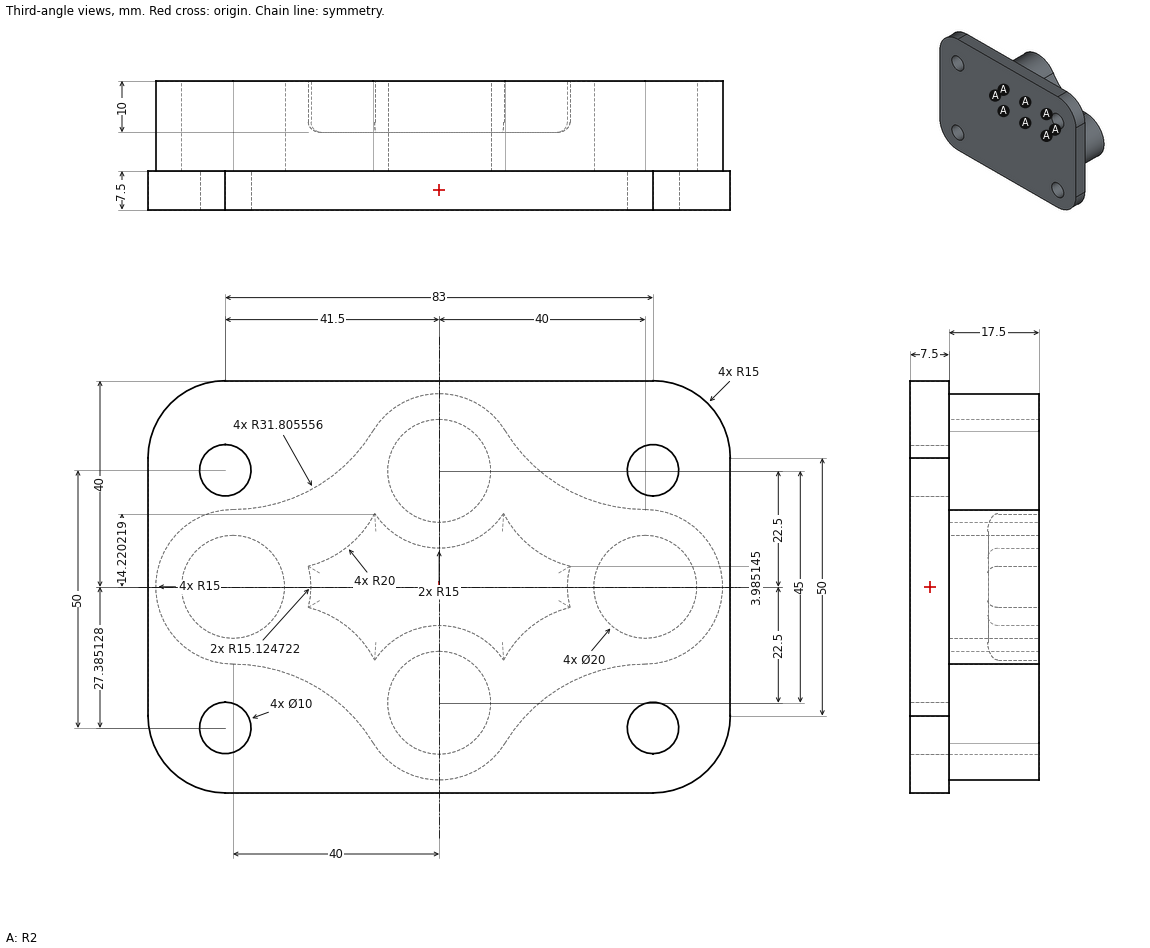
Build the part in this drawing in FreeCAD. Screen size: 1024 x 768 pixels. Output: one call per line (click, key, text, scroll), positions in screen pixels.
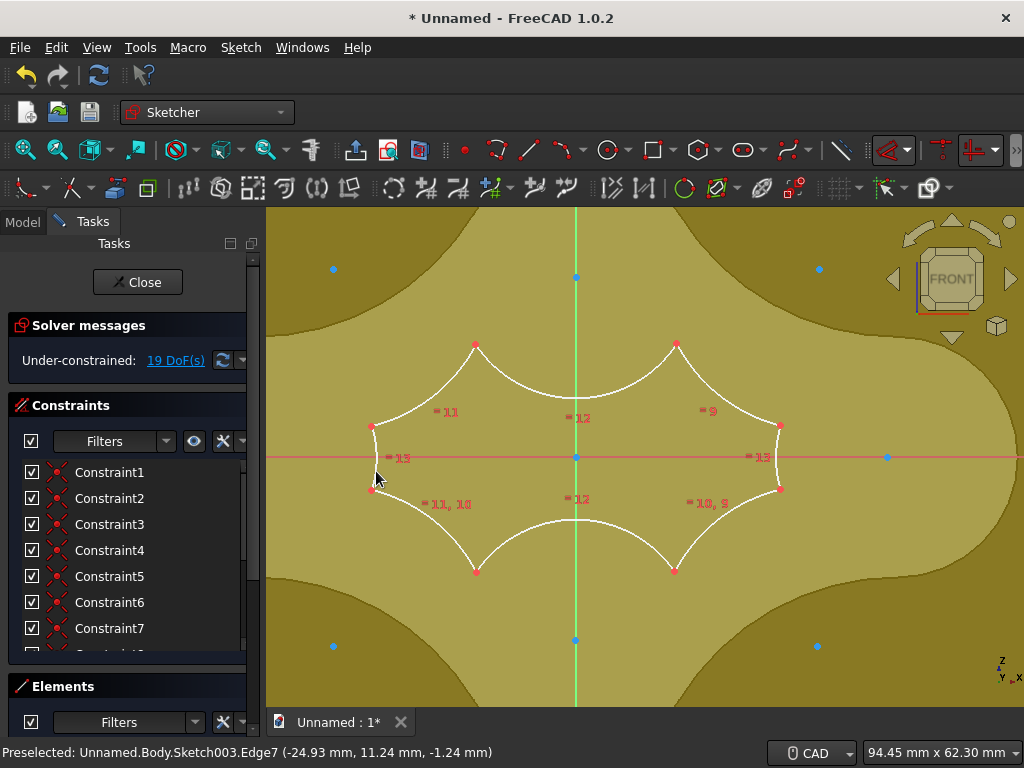
click(576, 278)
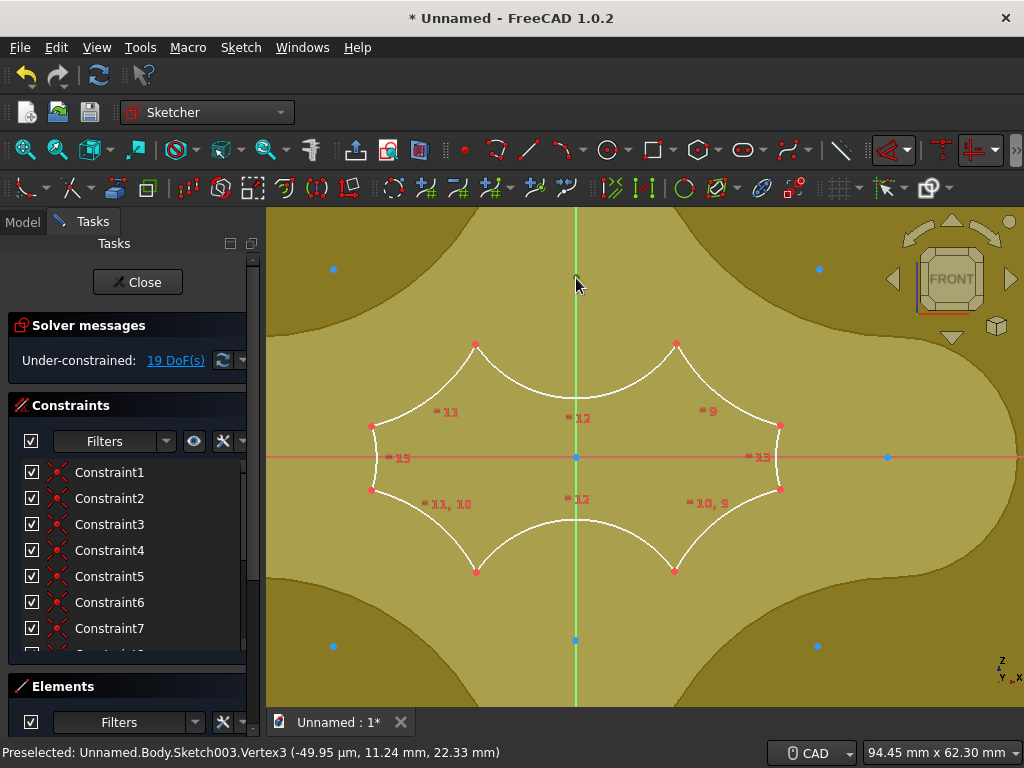
click(576, 647)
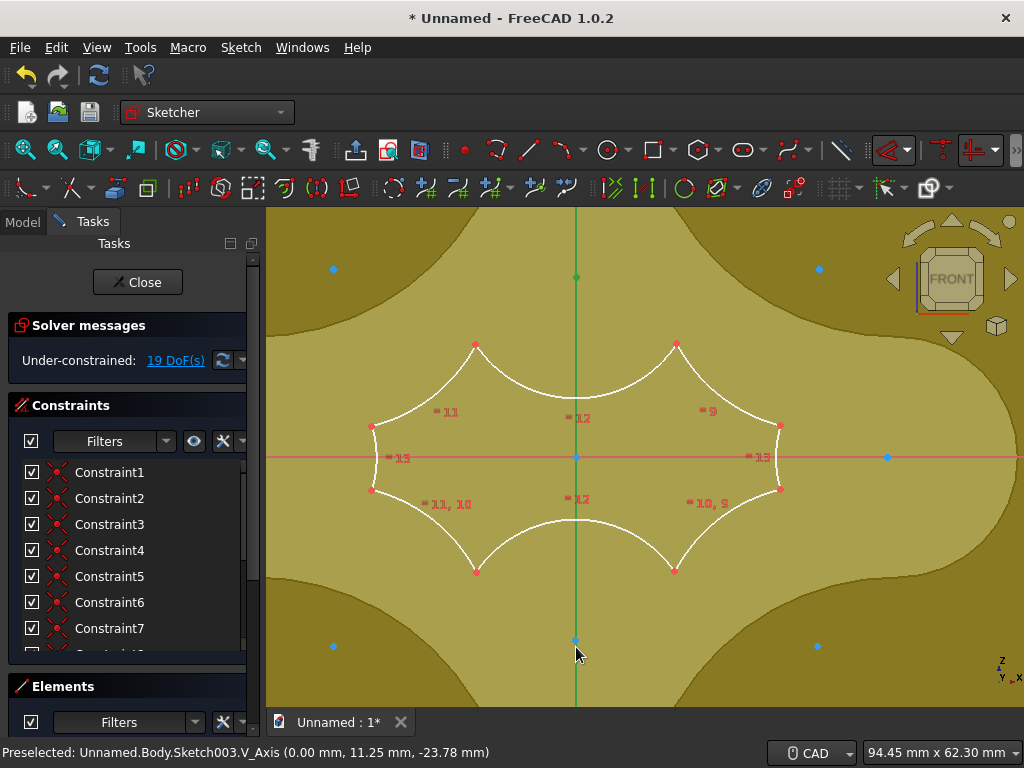
click(942, 150)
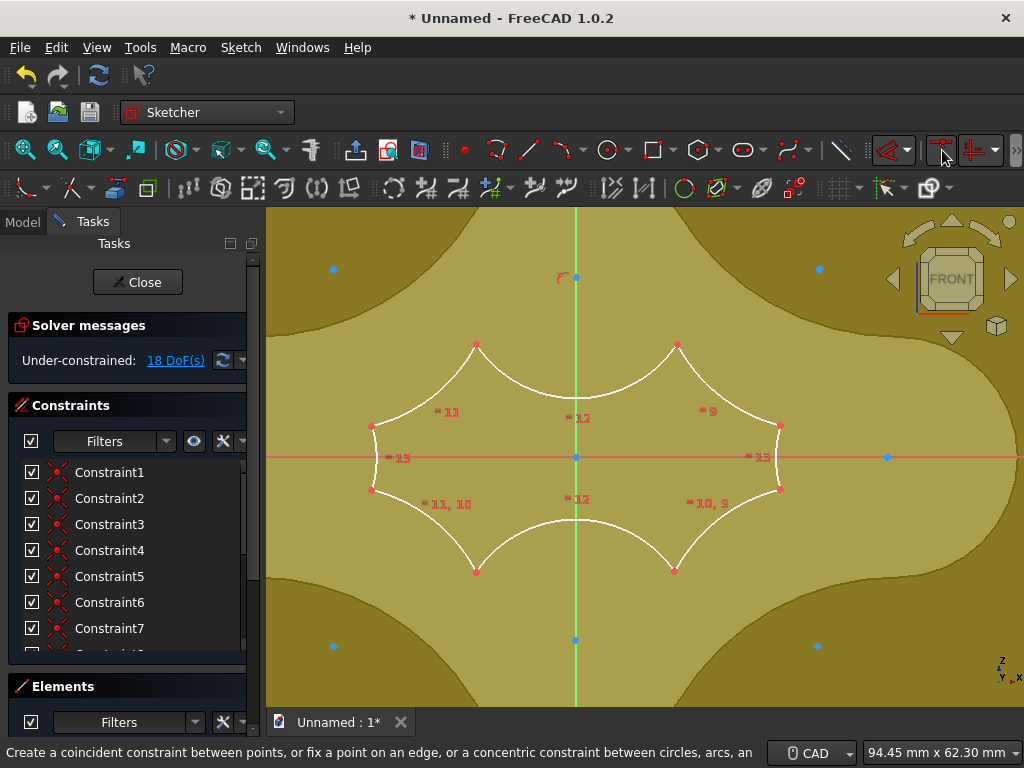
scroll(336, 456, down, 1)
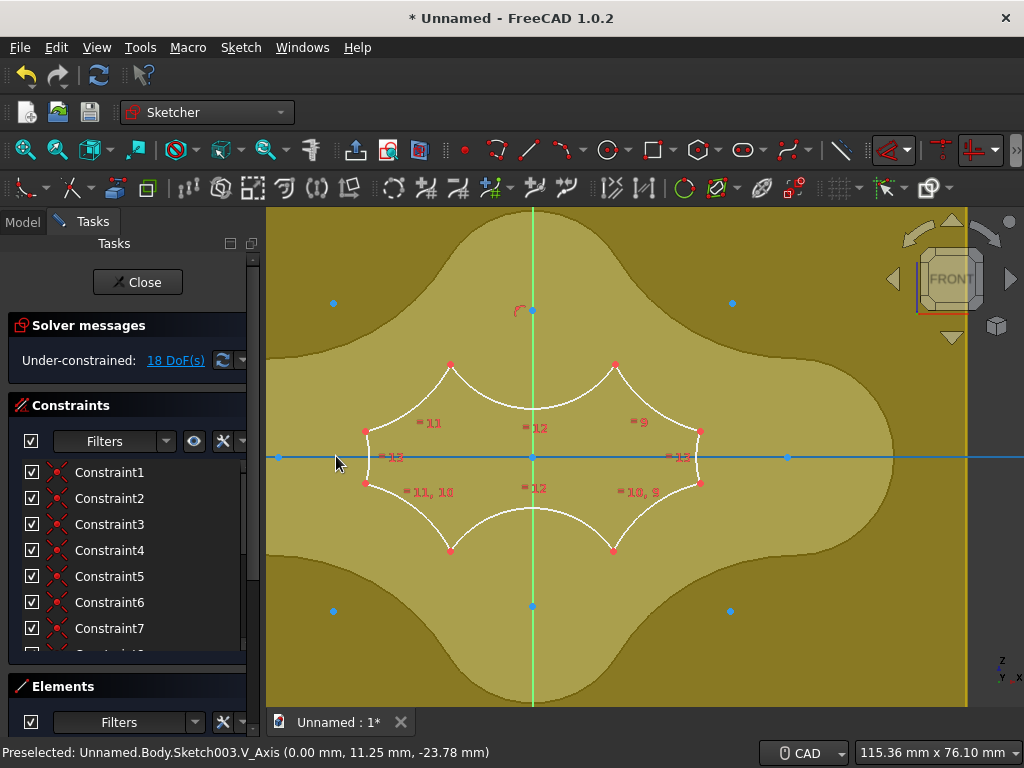
click(787, 458)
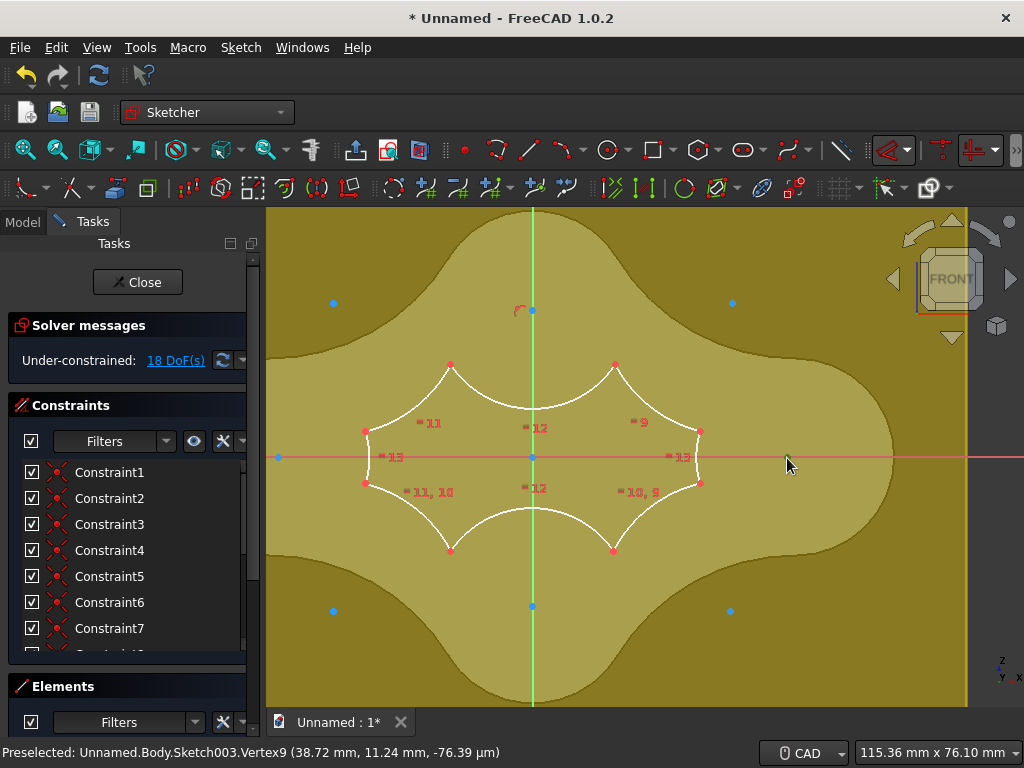
click(334, 457)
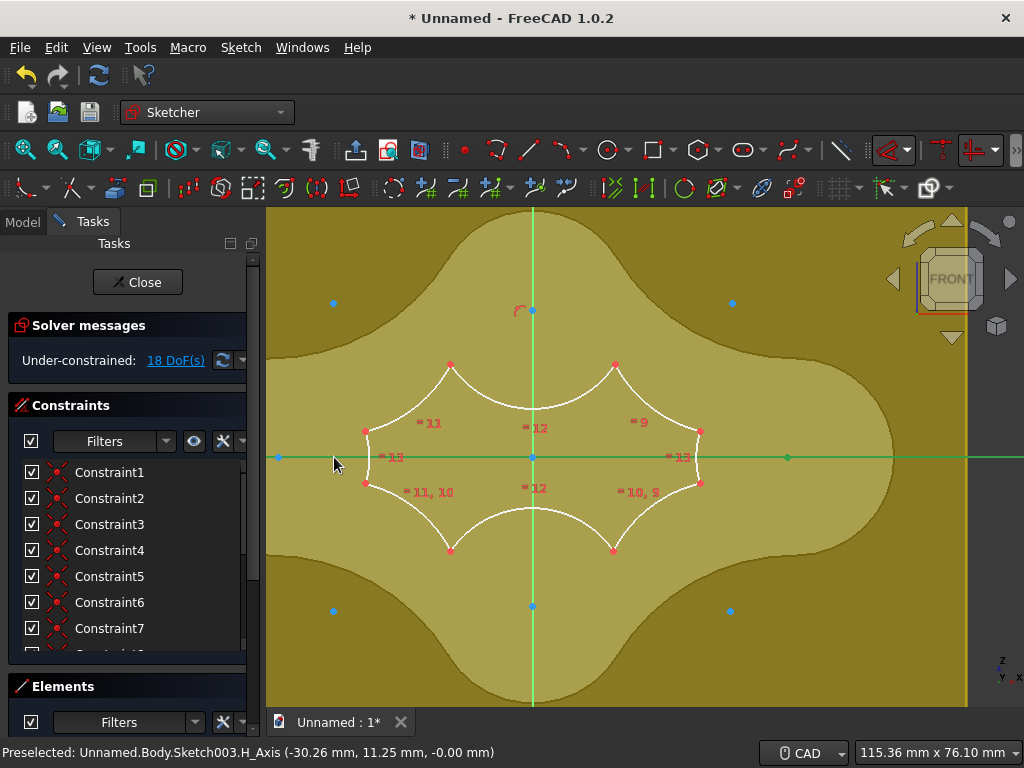
click(942, 150)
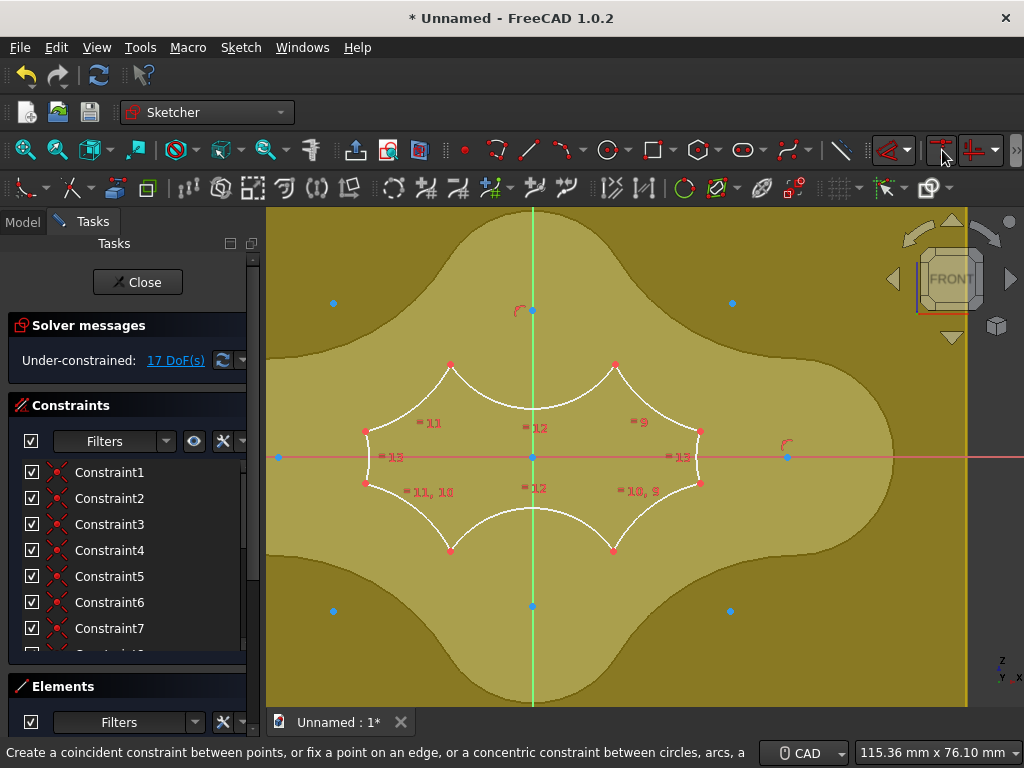
click(532, 607)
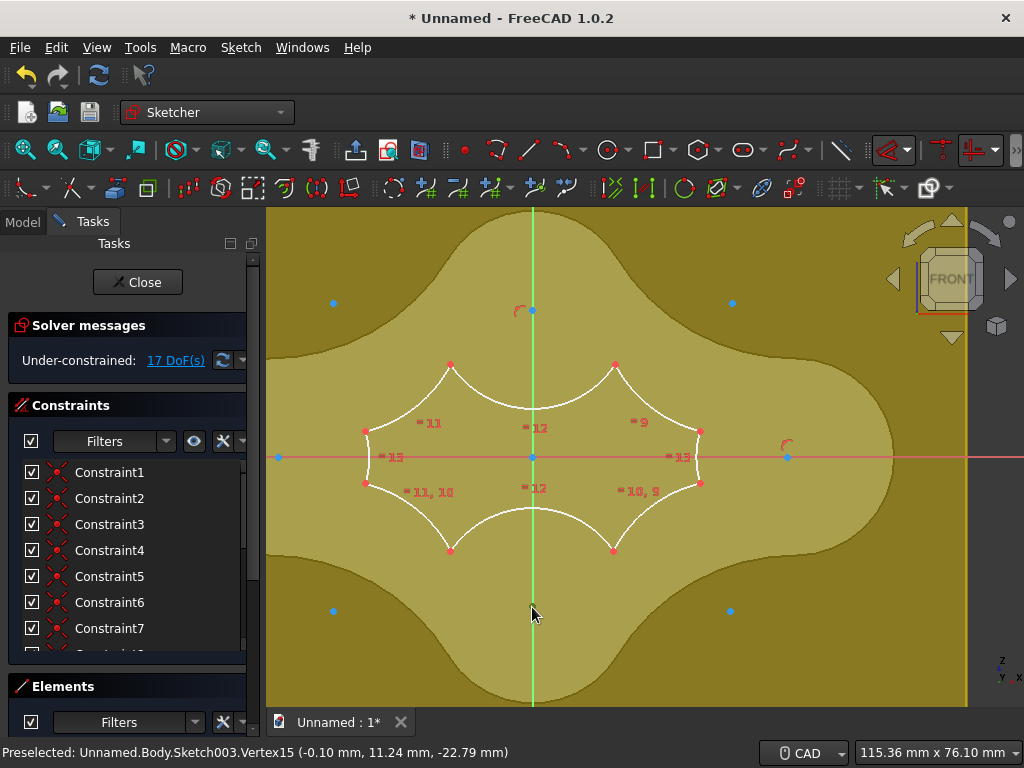
click(533, 647)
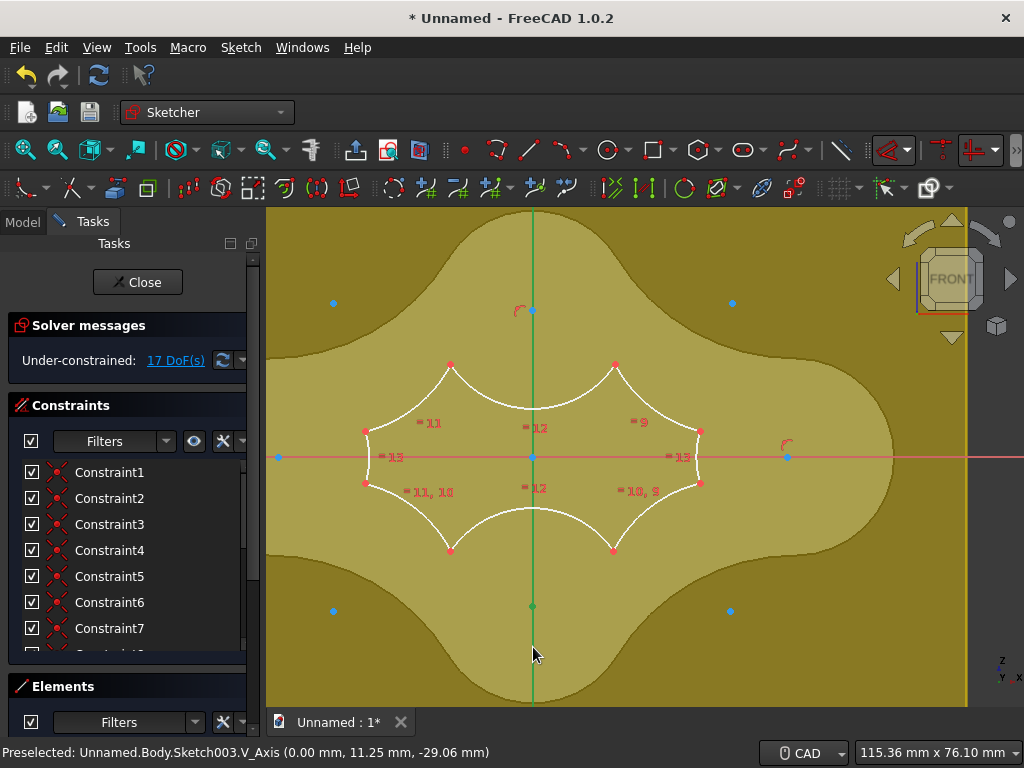
click(942, 150)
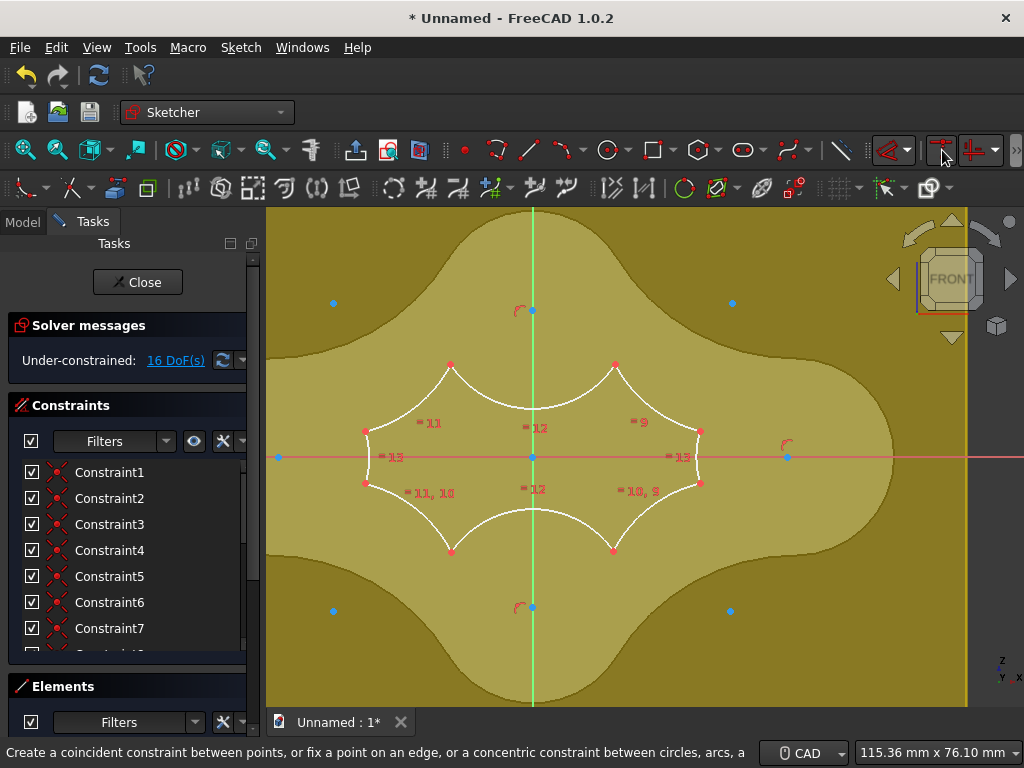
scroll(859, 457, down, 1)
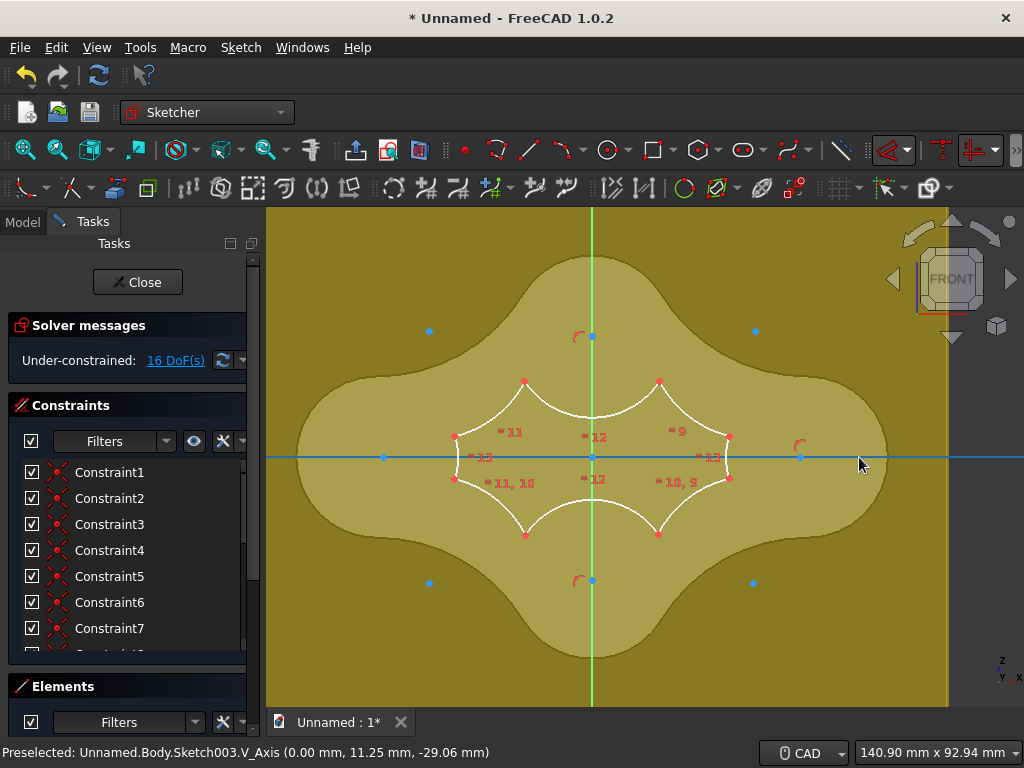
click(384, 458)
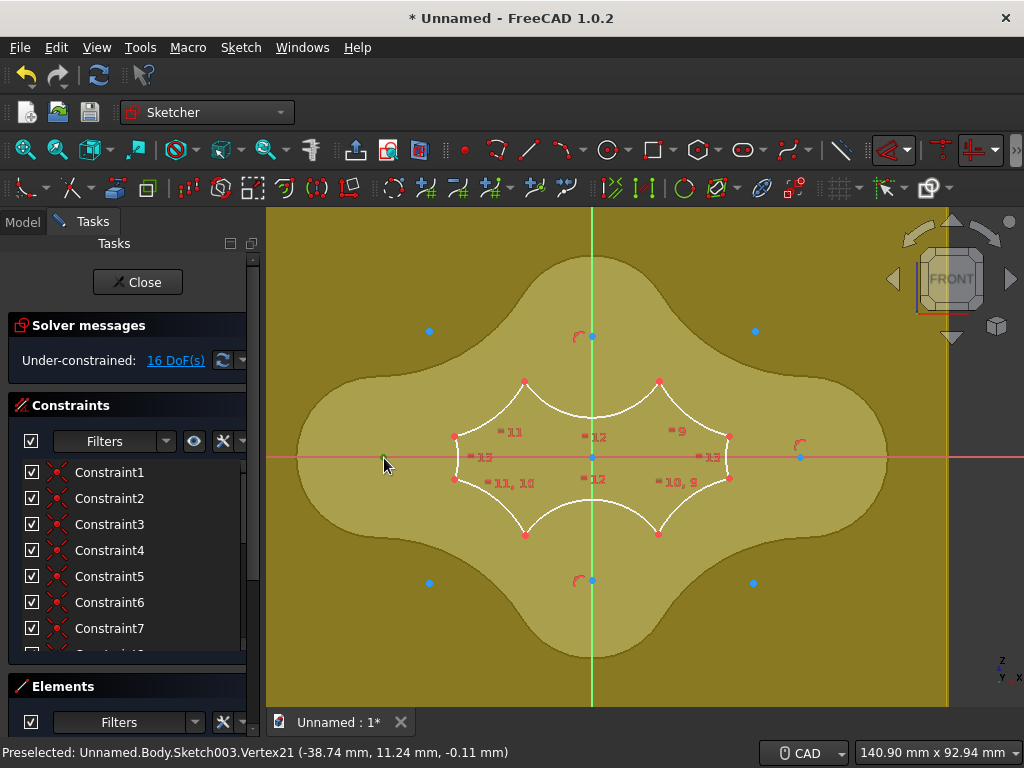
click(334, 457)